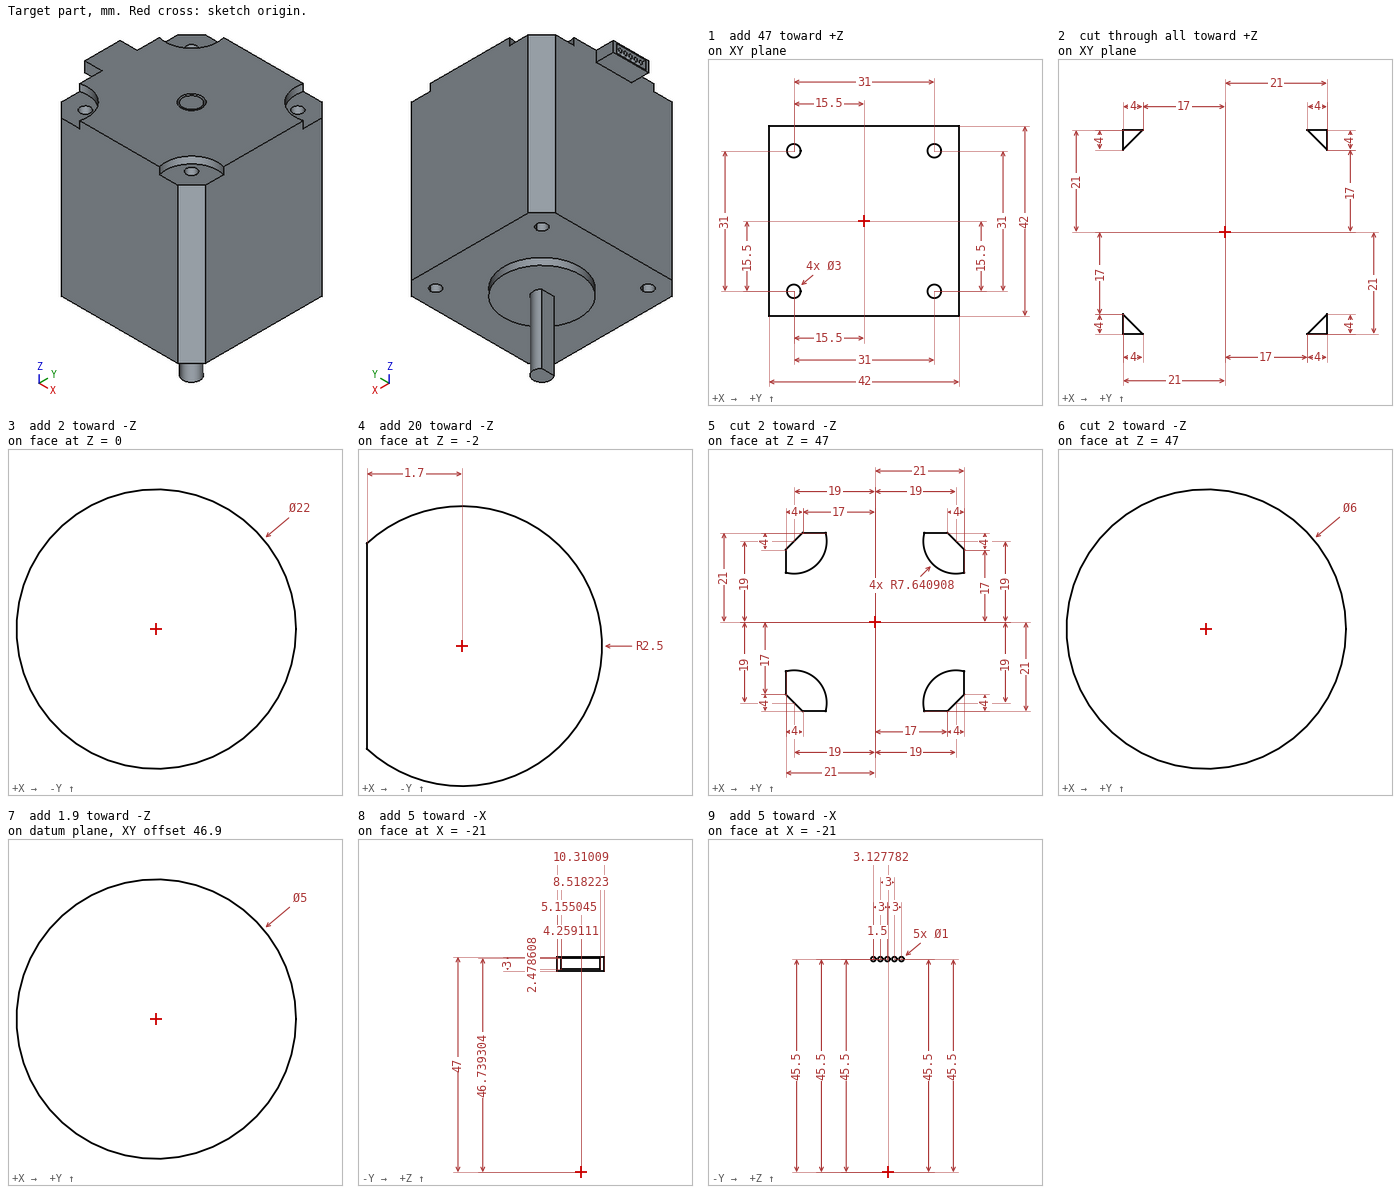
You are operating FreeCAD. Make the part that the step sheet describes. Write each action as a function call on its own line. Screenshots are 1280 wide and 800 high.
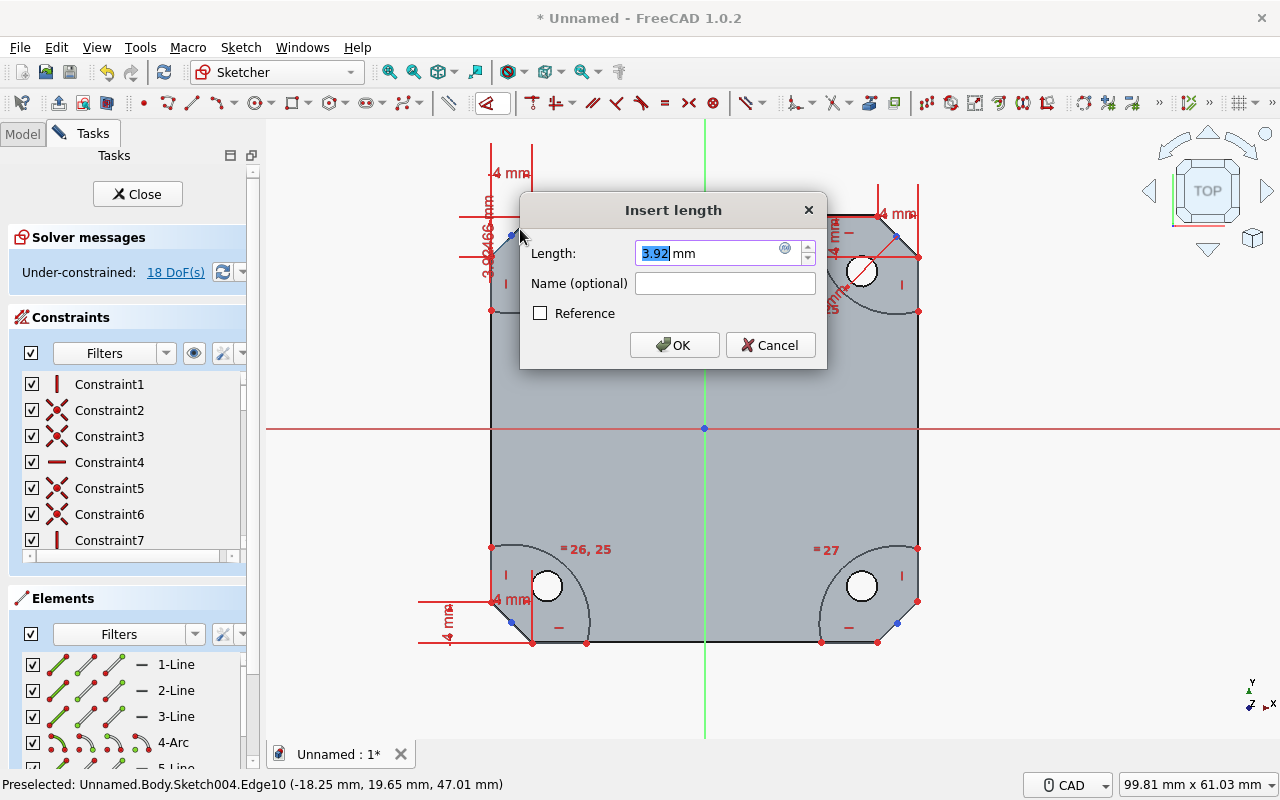
text(4)
key(Return)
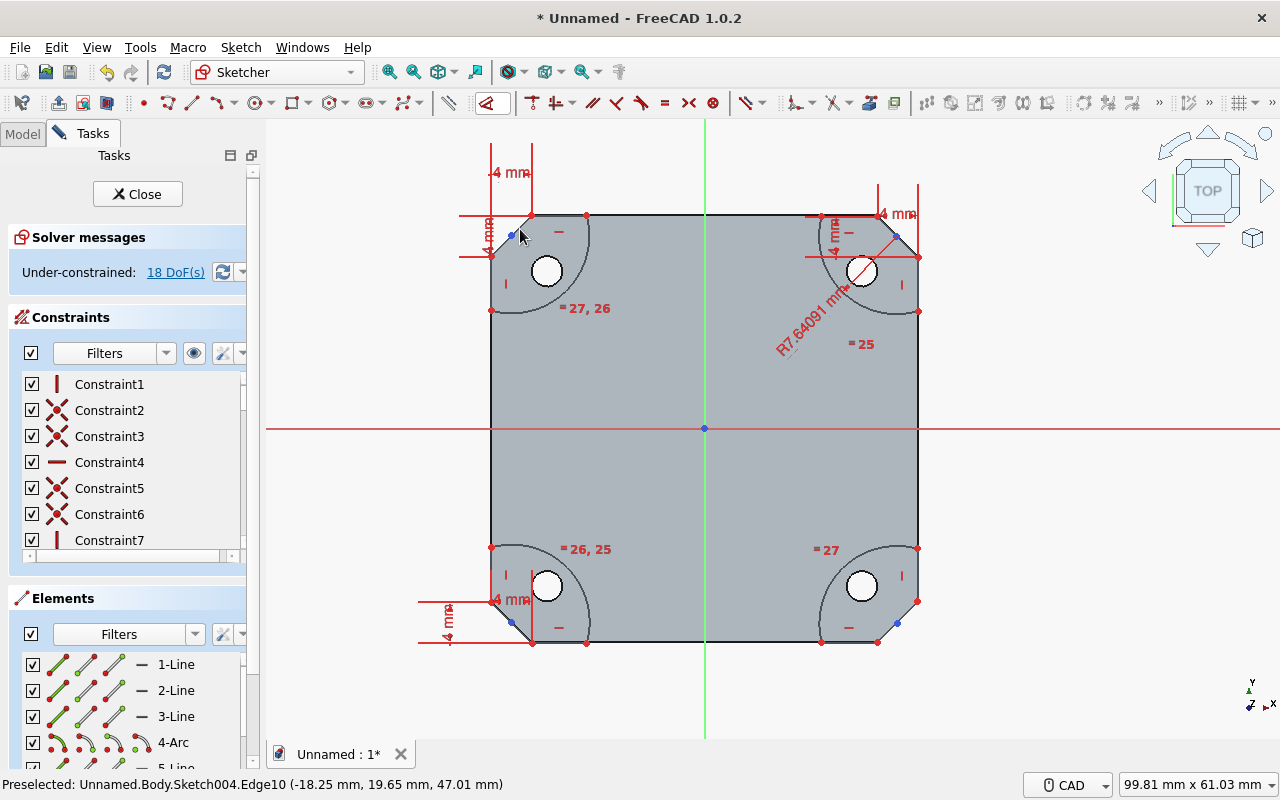
click(889, 631)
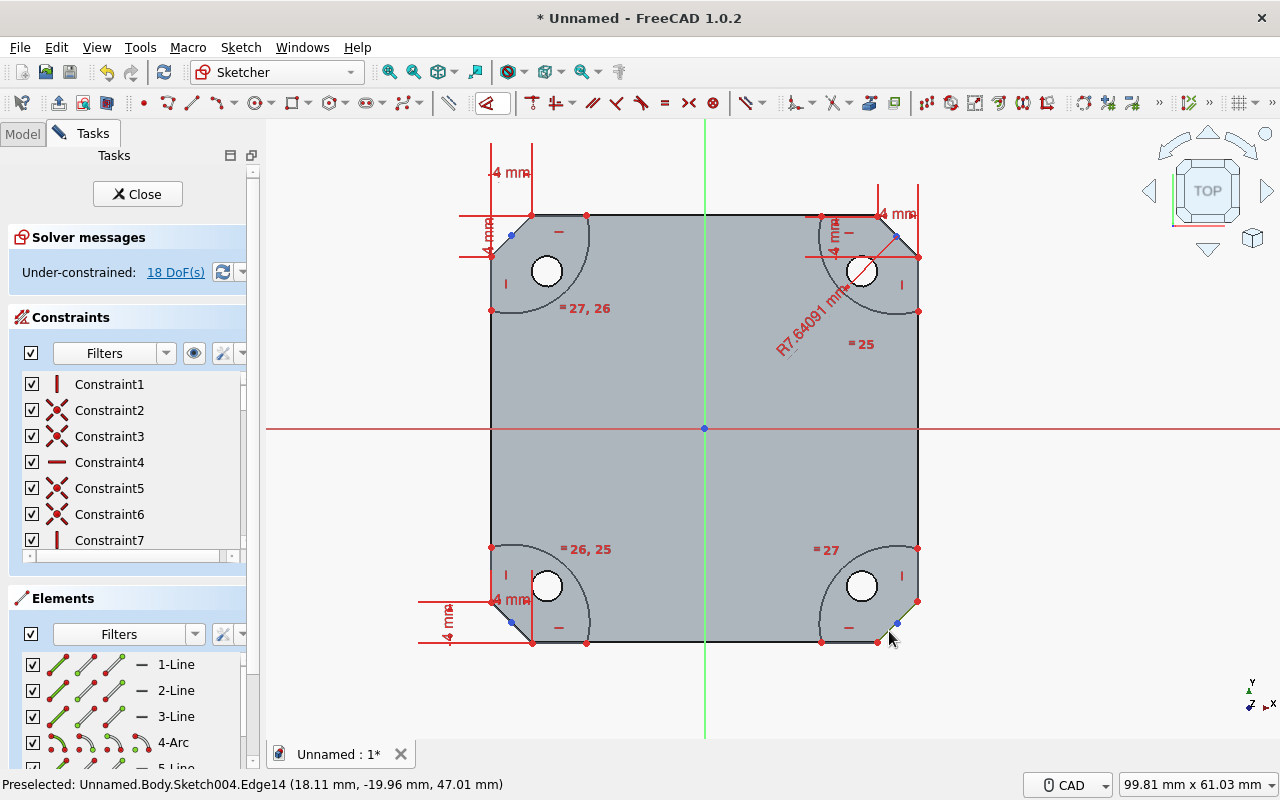
click(504, 104)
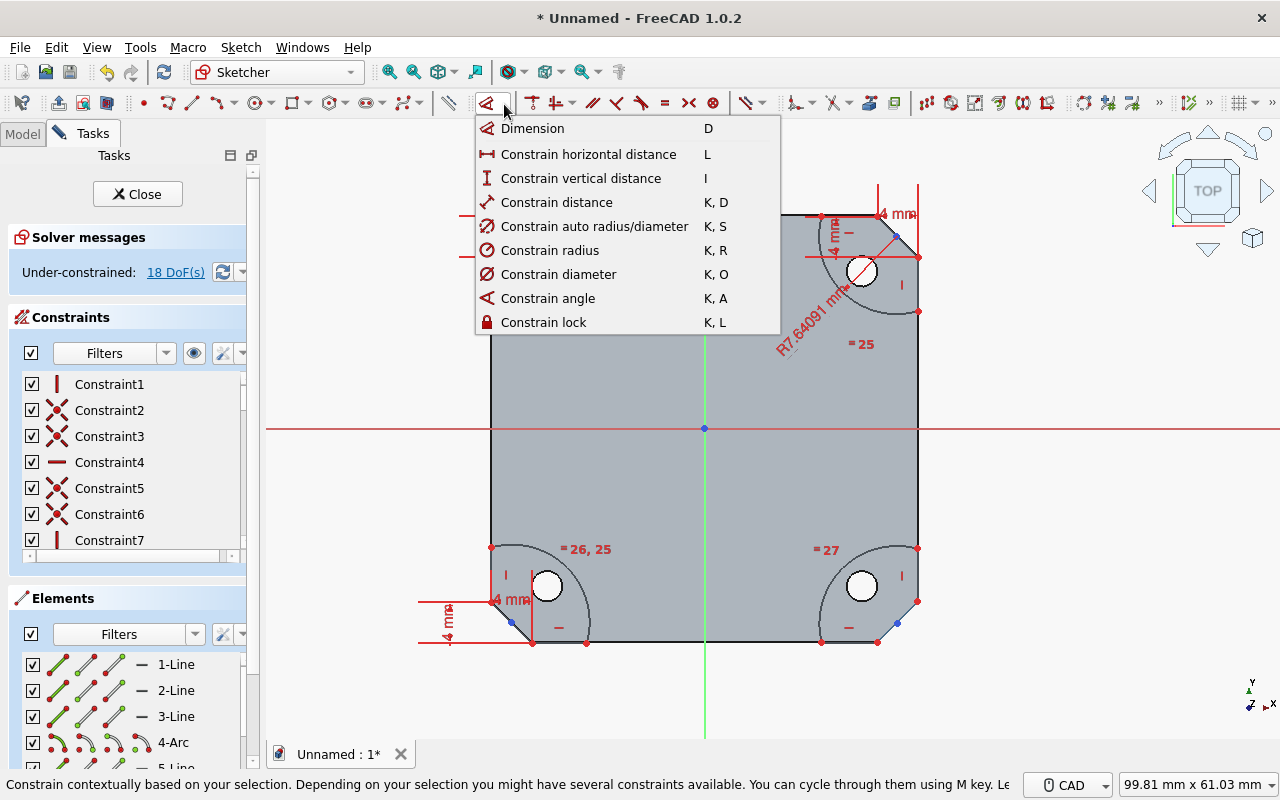
click(628, 154)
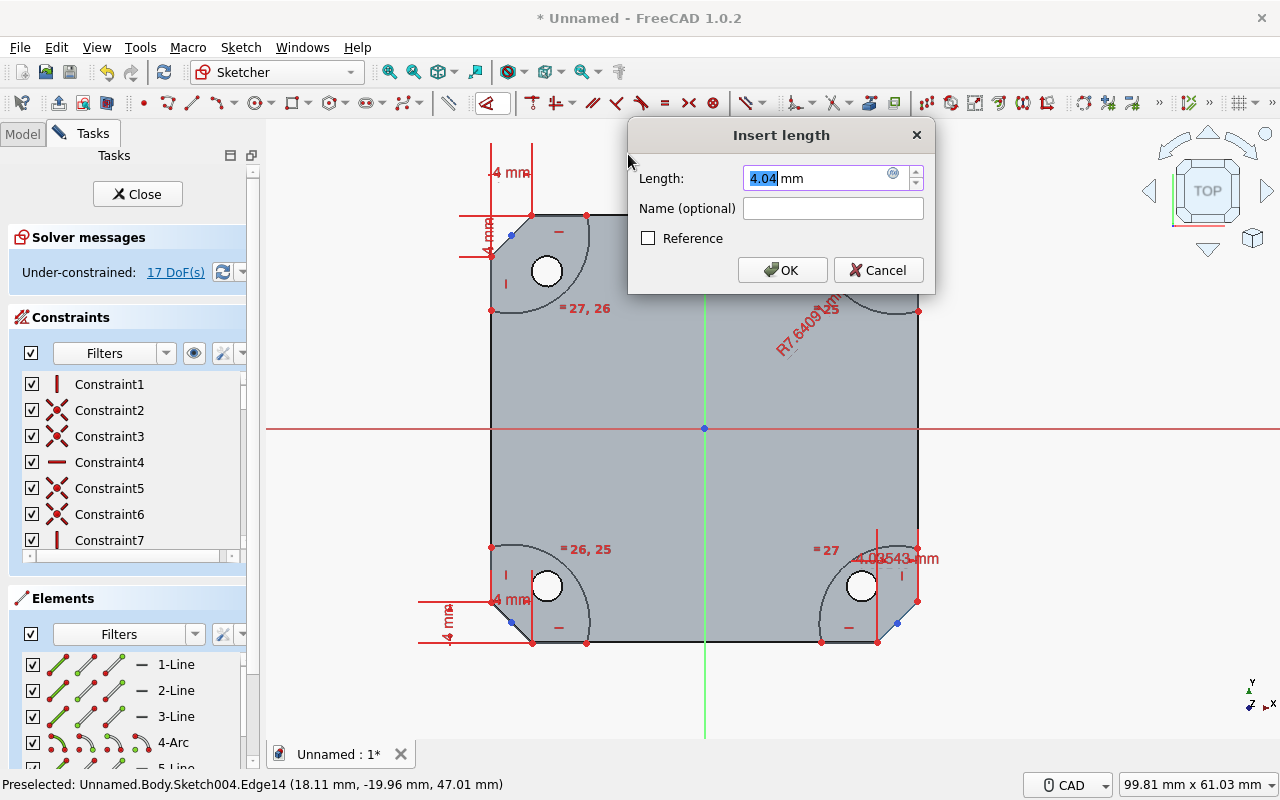
text(4)
key(Return)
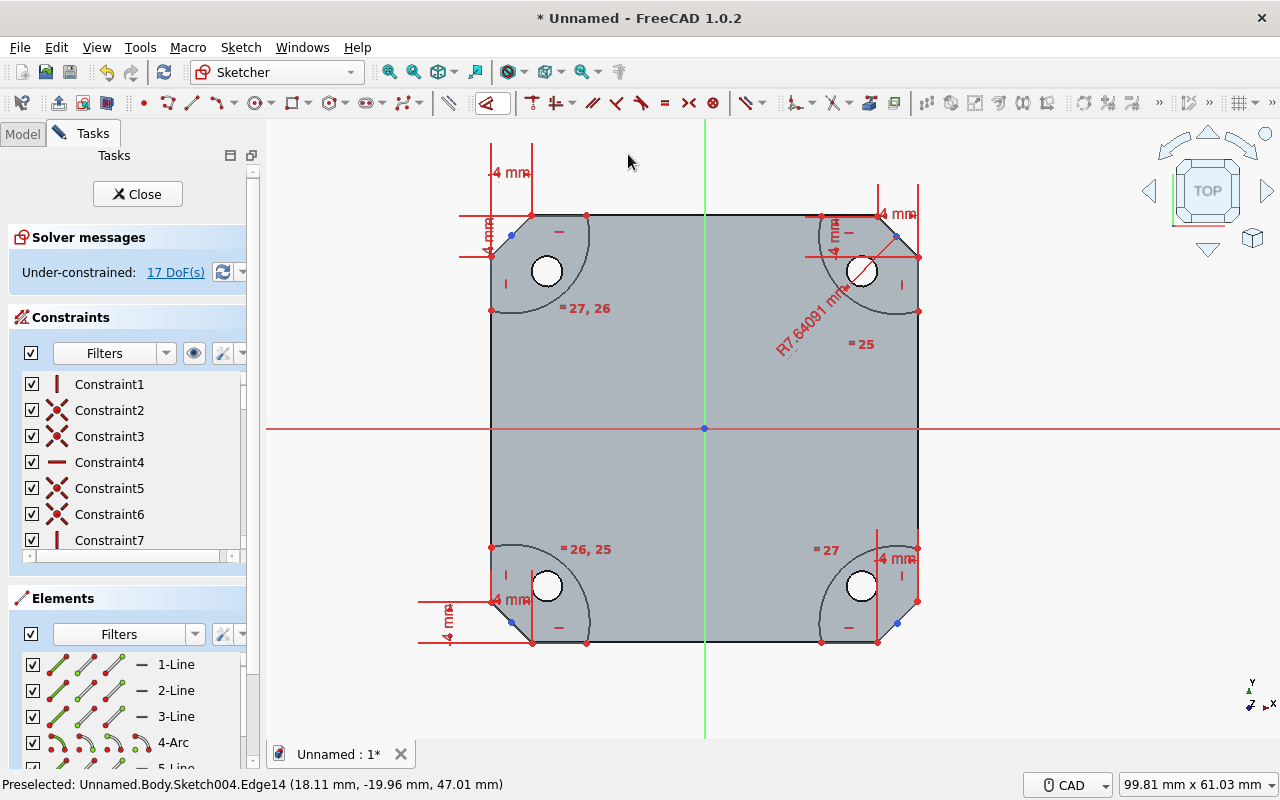
click(889, 631)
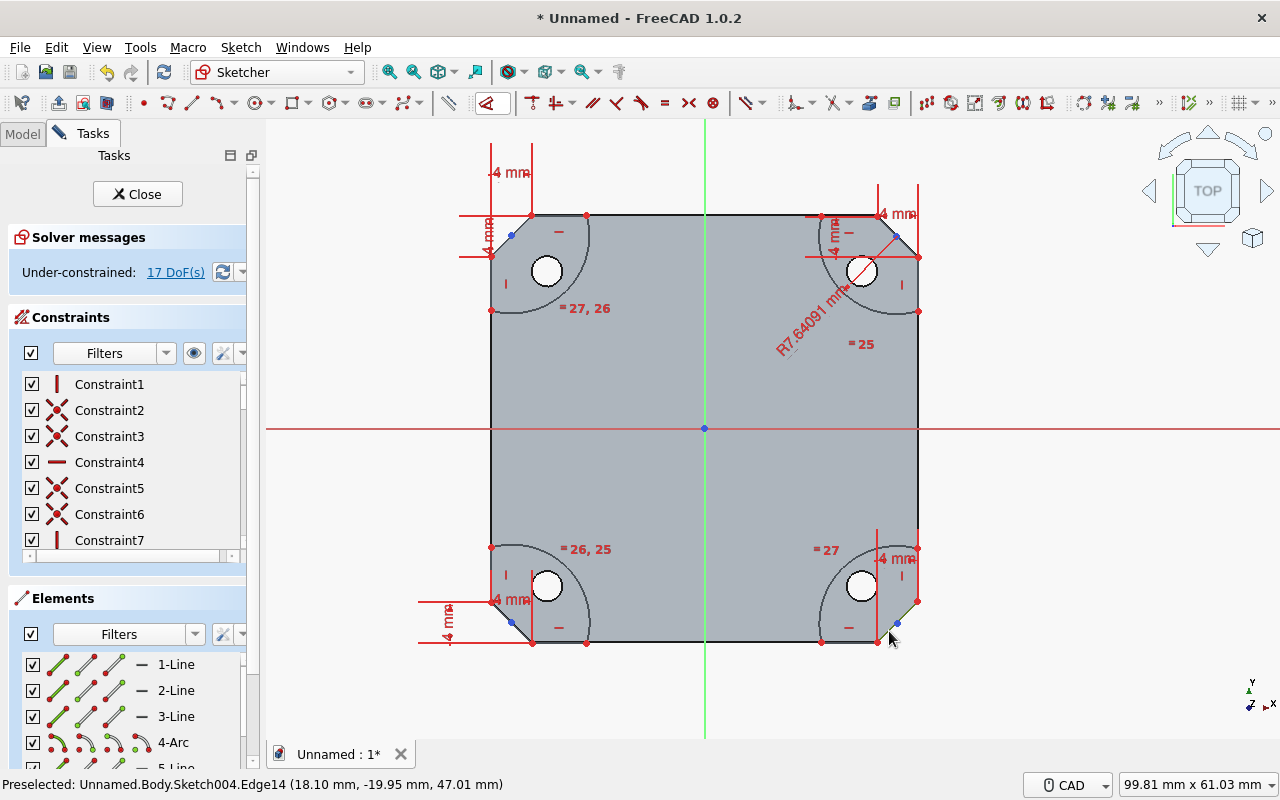
click(504, 104)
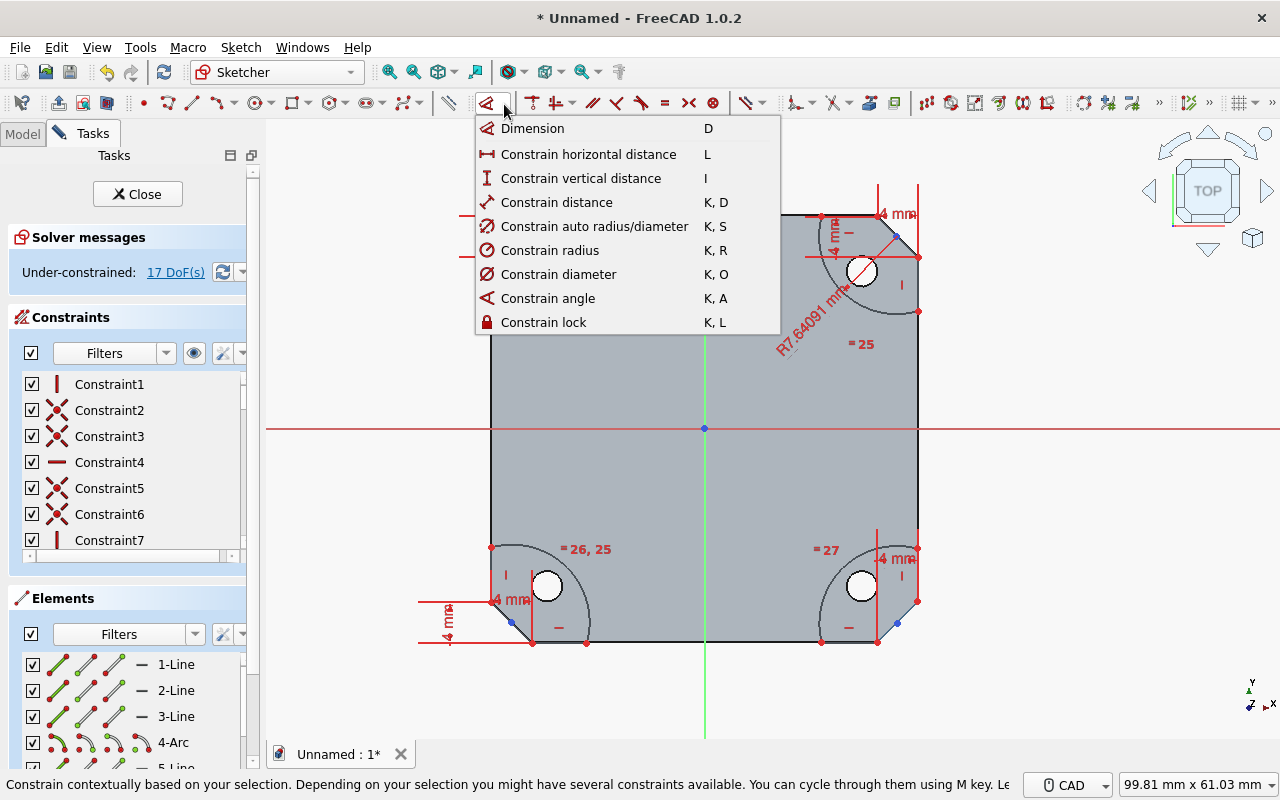
click(628, 178)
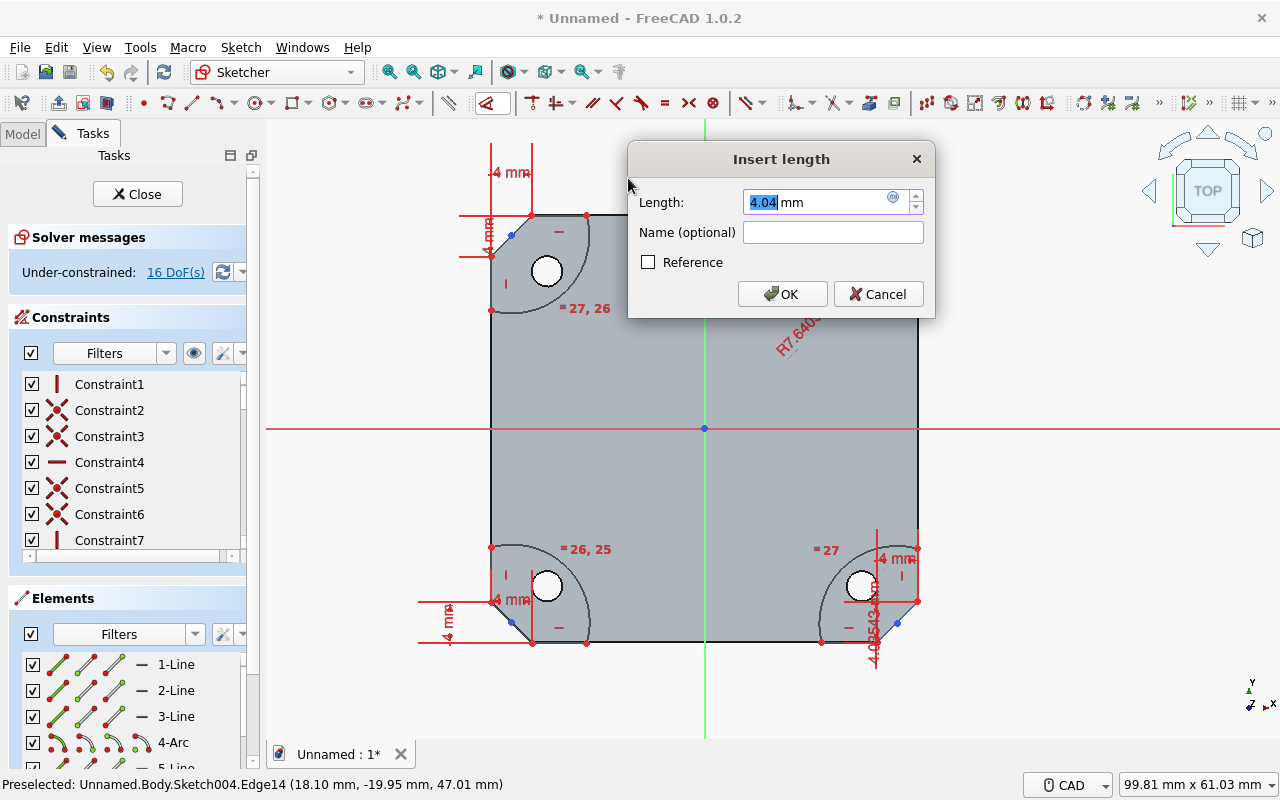
text(4)
key(Return)